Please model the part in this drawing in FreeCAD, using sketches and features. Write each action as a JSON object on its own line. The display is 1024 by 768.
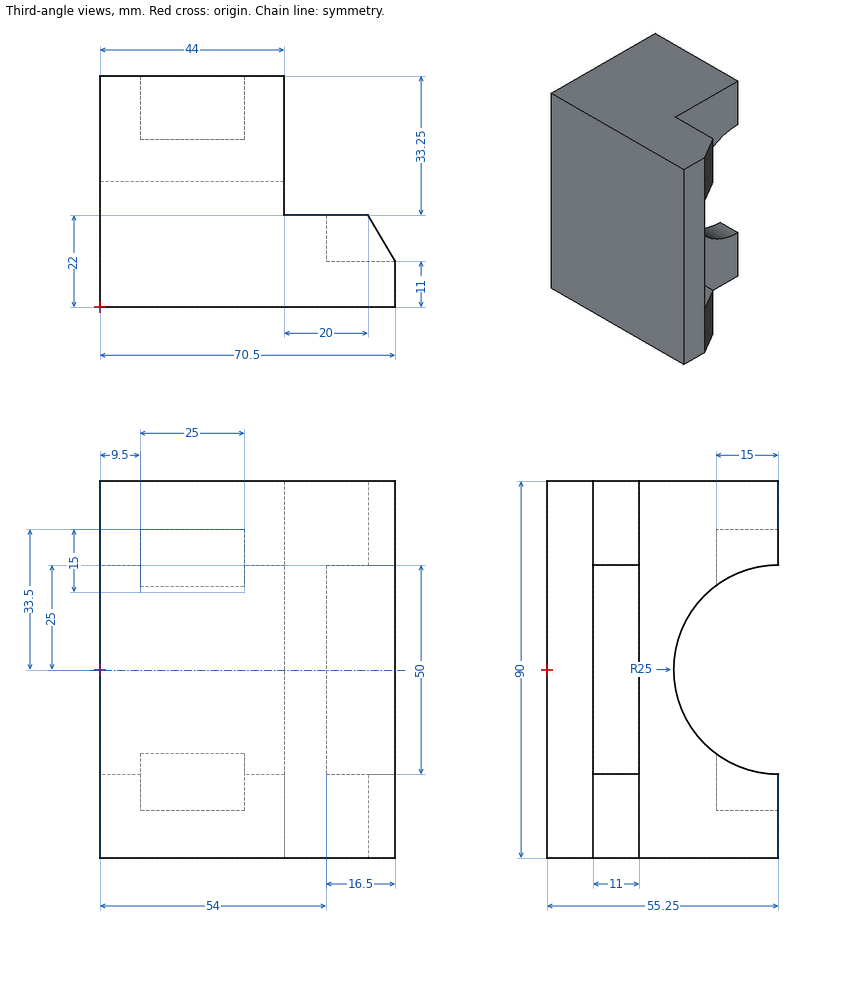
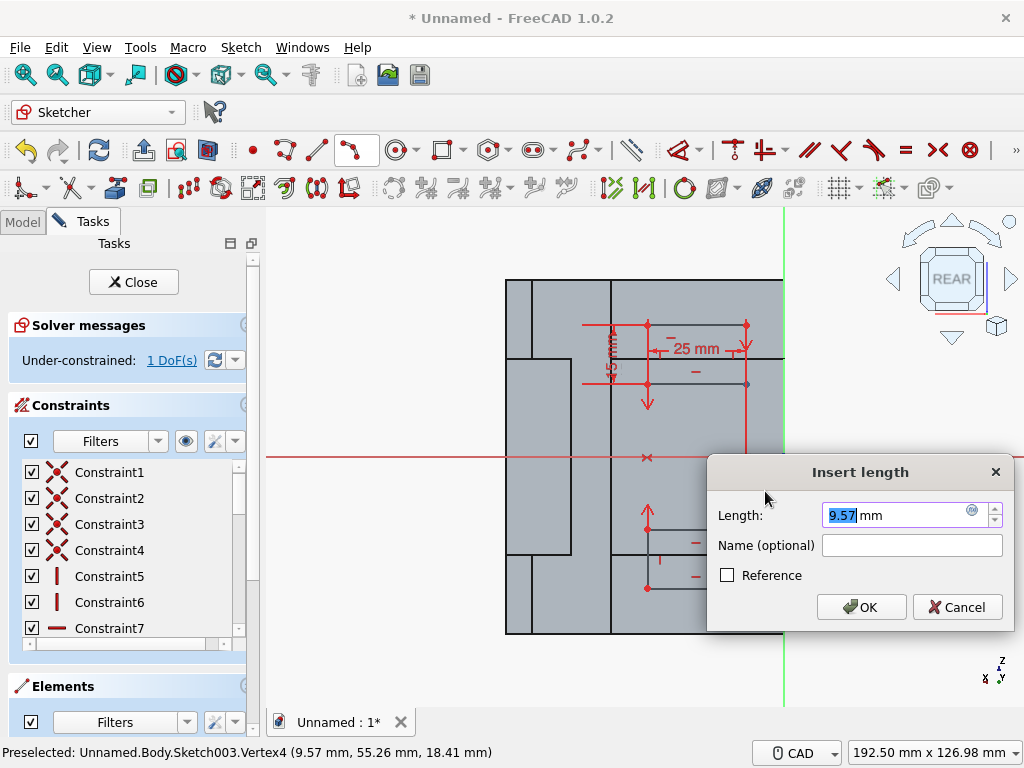
{"action": "type", "text": "9.5"}
{"action": "key", "text": "Return"}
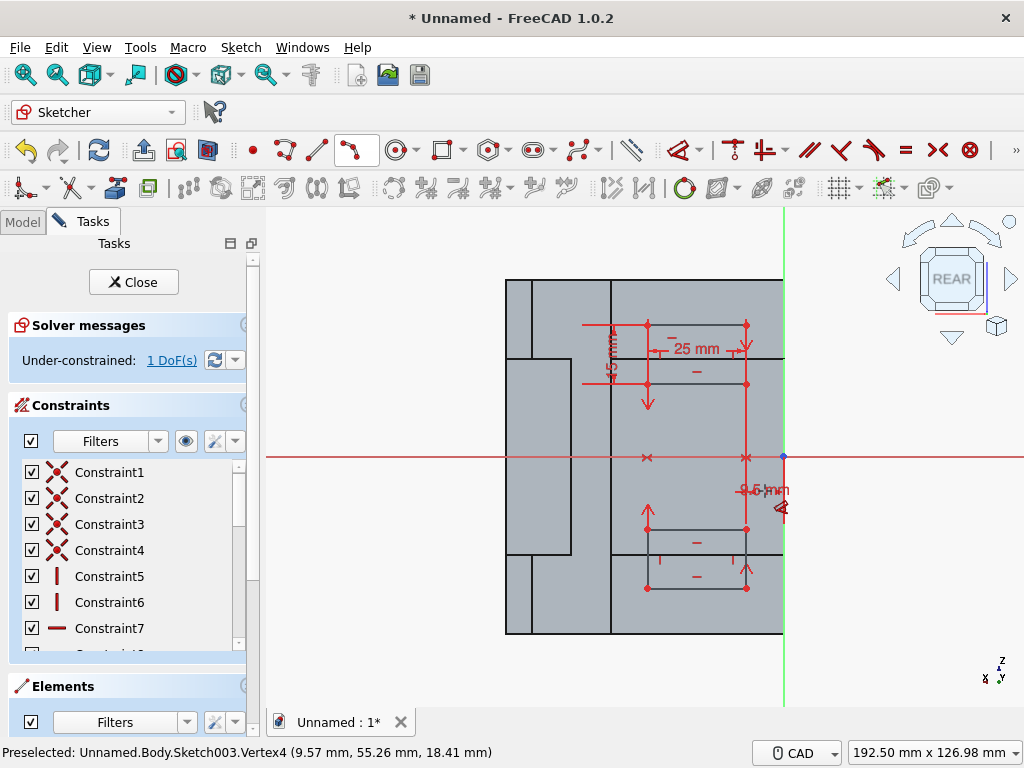
{"action": "left_click", "coordinate": [648, 325]}
{"action": "left_click", "coordinate": [818, 391]}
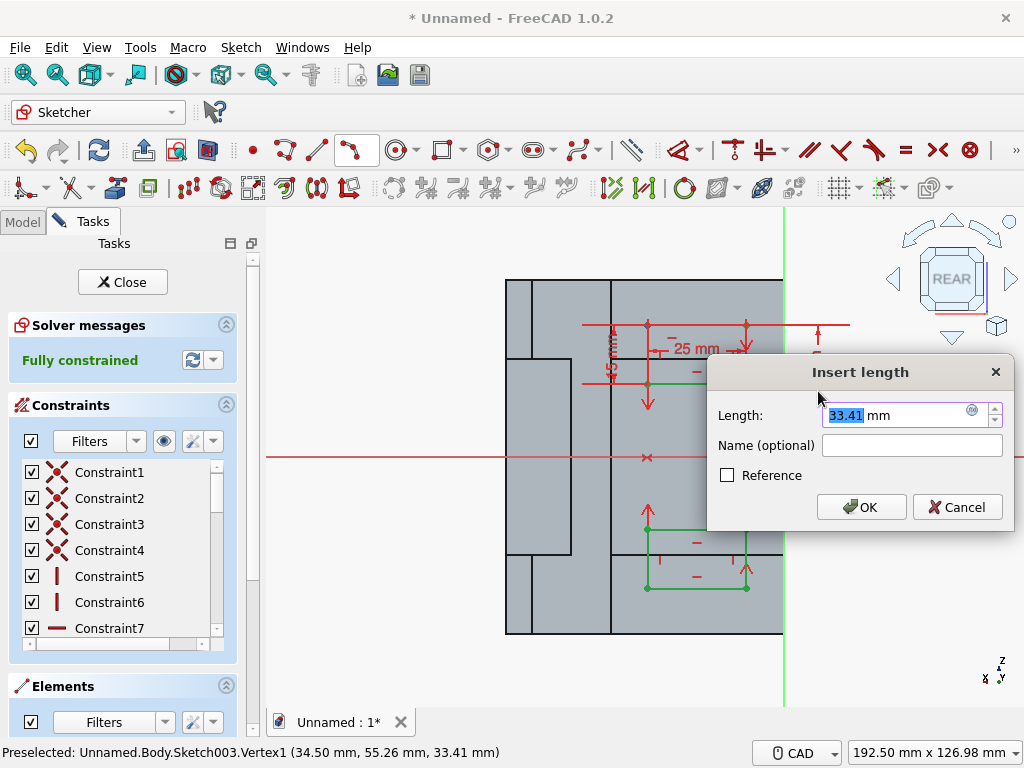
{"action": "type", "text": "33.5"}
{"action": "key", "text": "Return"}
{"action": "key", "text": "Escape"}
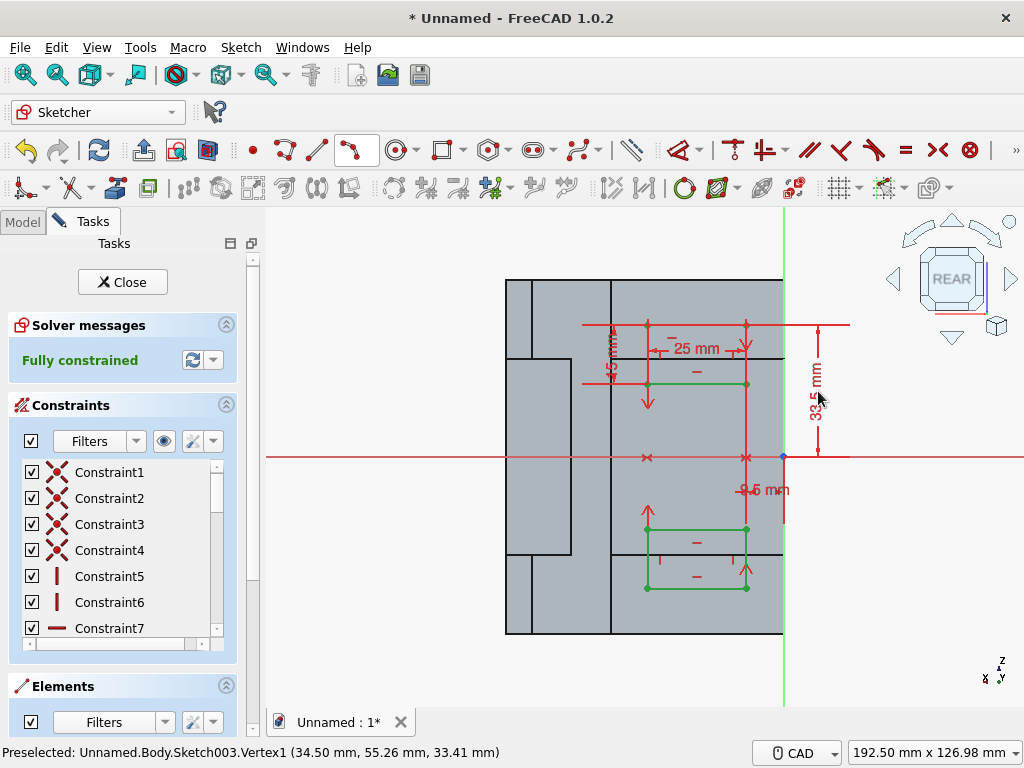
{"action": "left_click", "coordinate": [123, 282]}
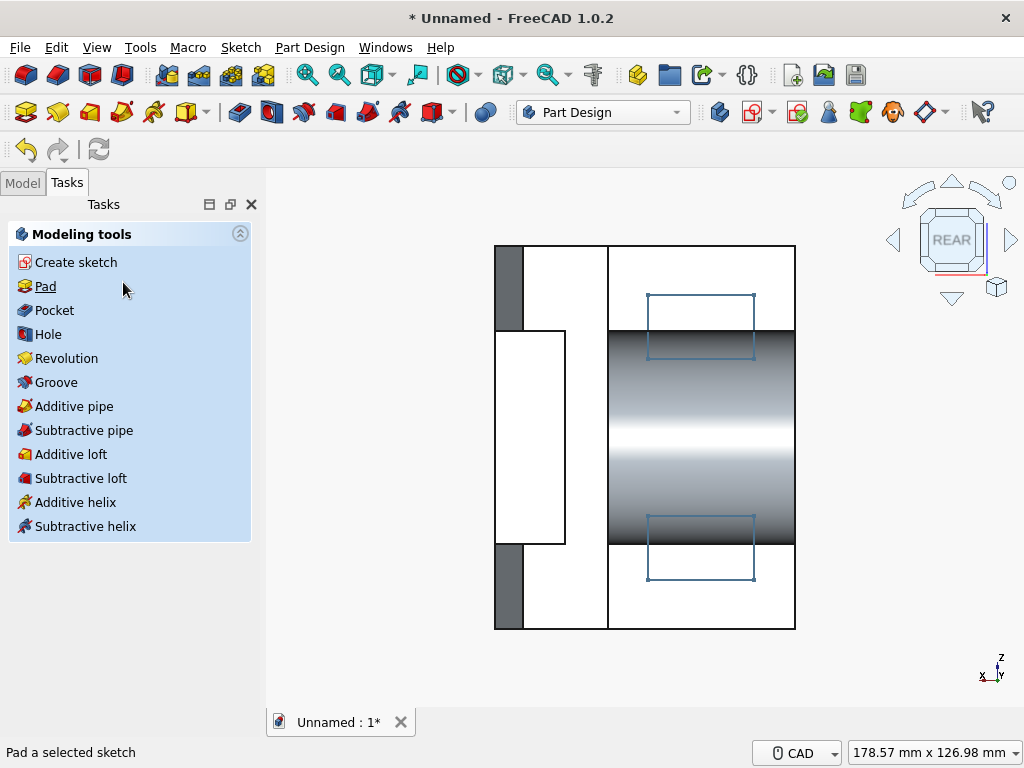
{"action": "left_click", "coordinate": [240, 112]}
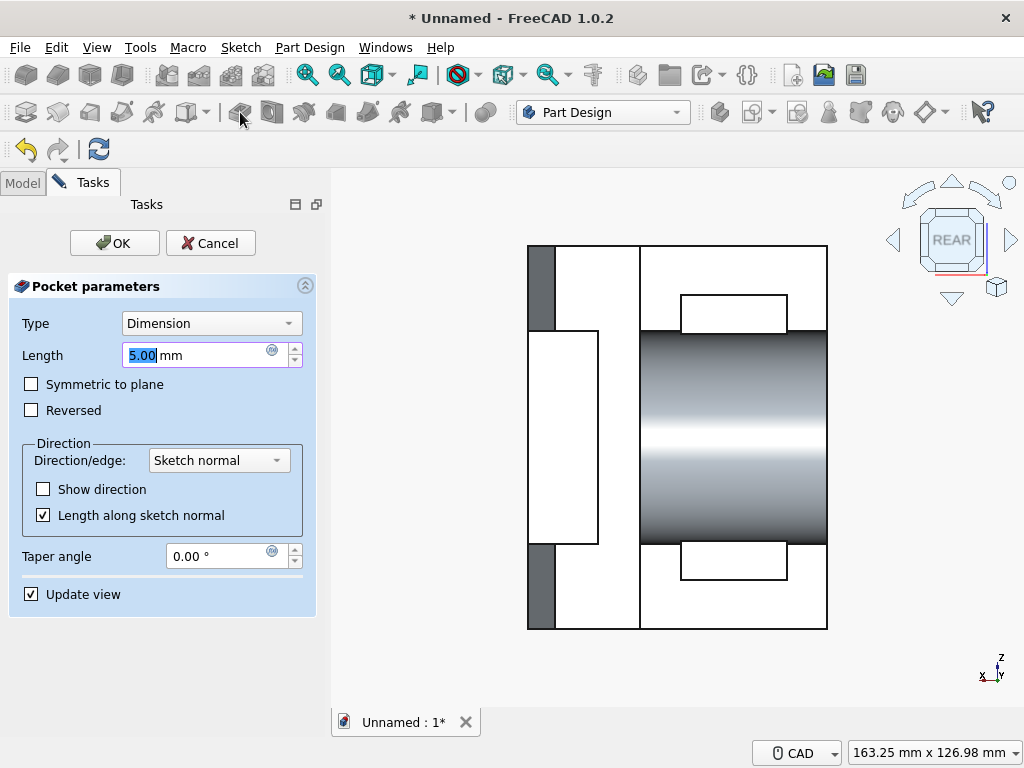
{"action": "type", "text": "15"}
{"action": "key", "text": "Tab"}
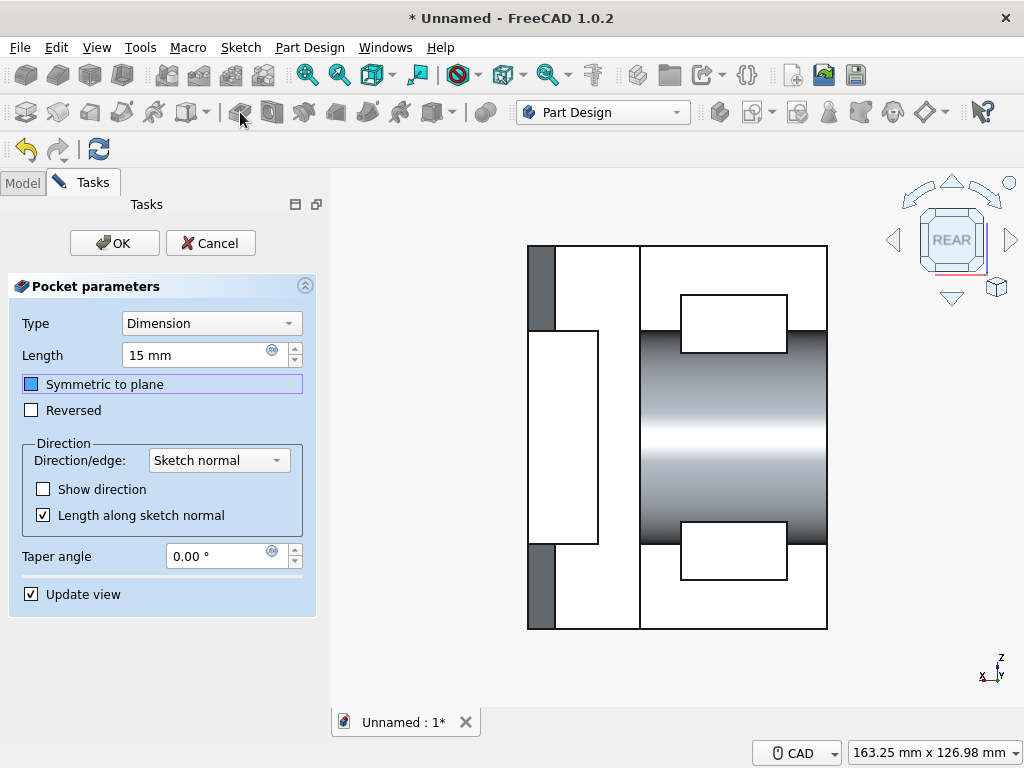
{"action": "left_click", "coordinate": [115, 243]}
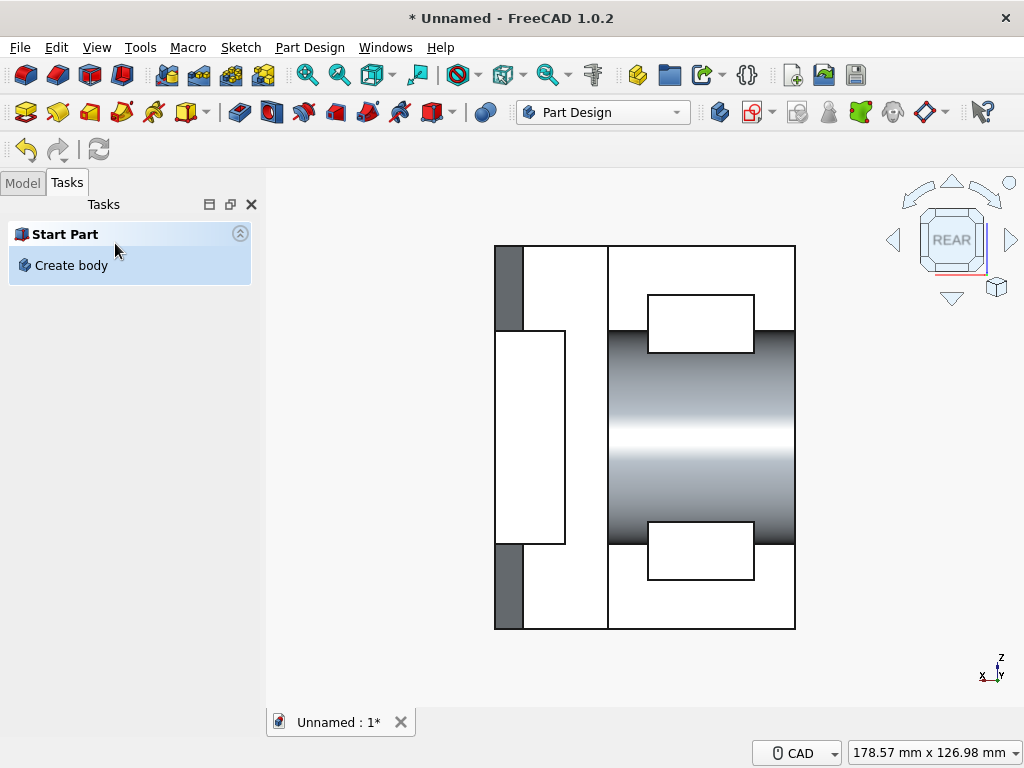
{"action": "key", "text": "0"}